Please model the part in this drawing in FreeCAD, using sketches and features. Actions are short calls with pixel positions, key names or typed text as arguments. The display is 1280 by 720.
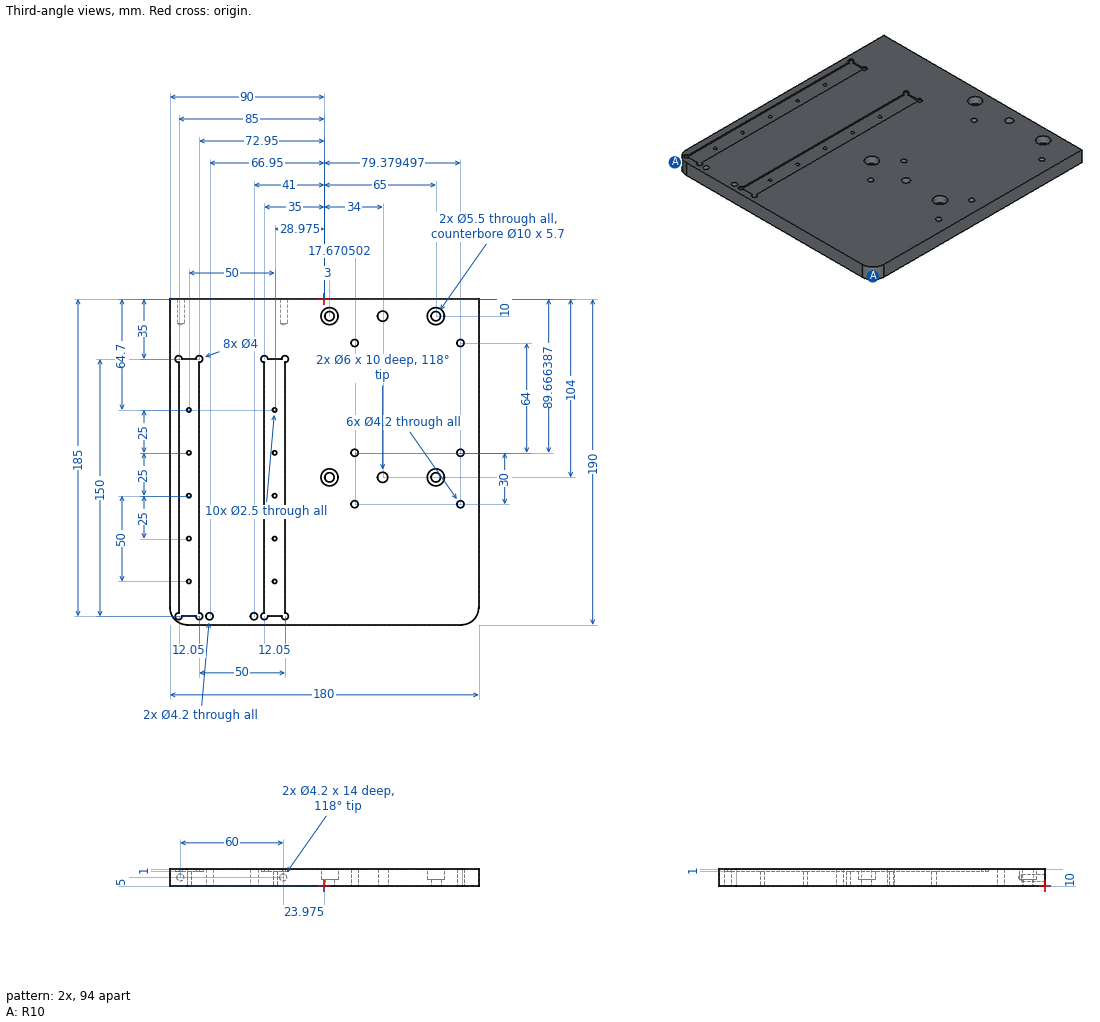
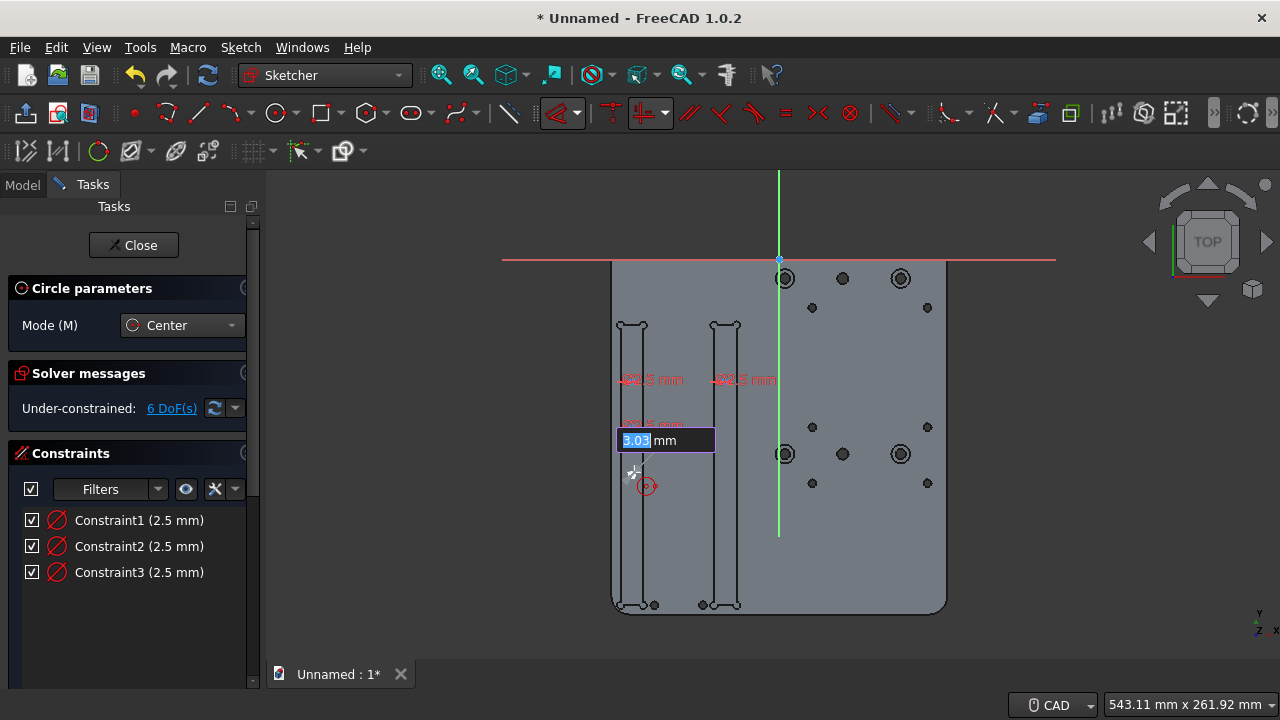
text(2.5)
key(Return)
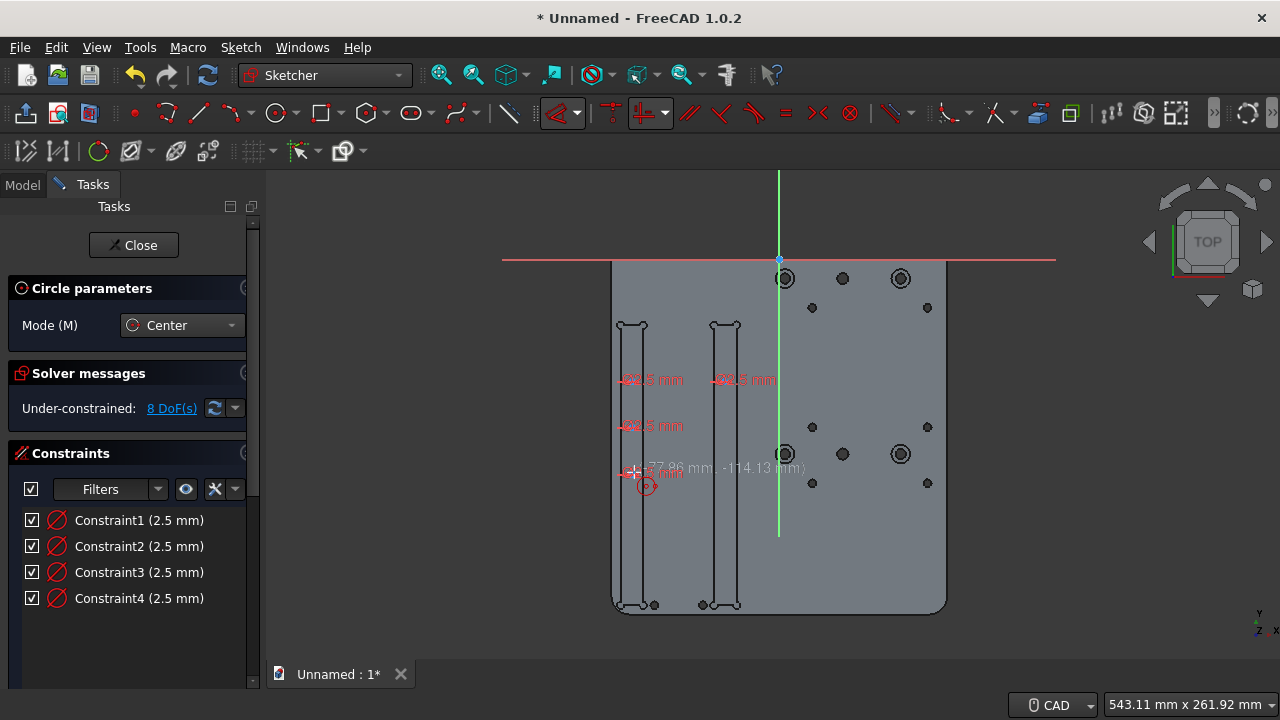
scroll(632, 567, up, 12)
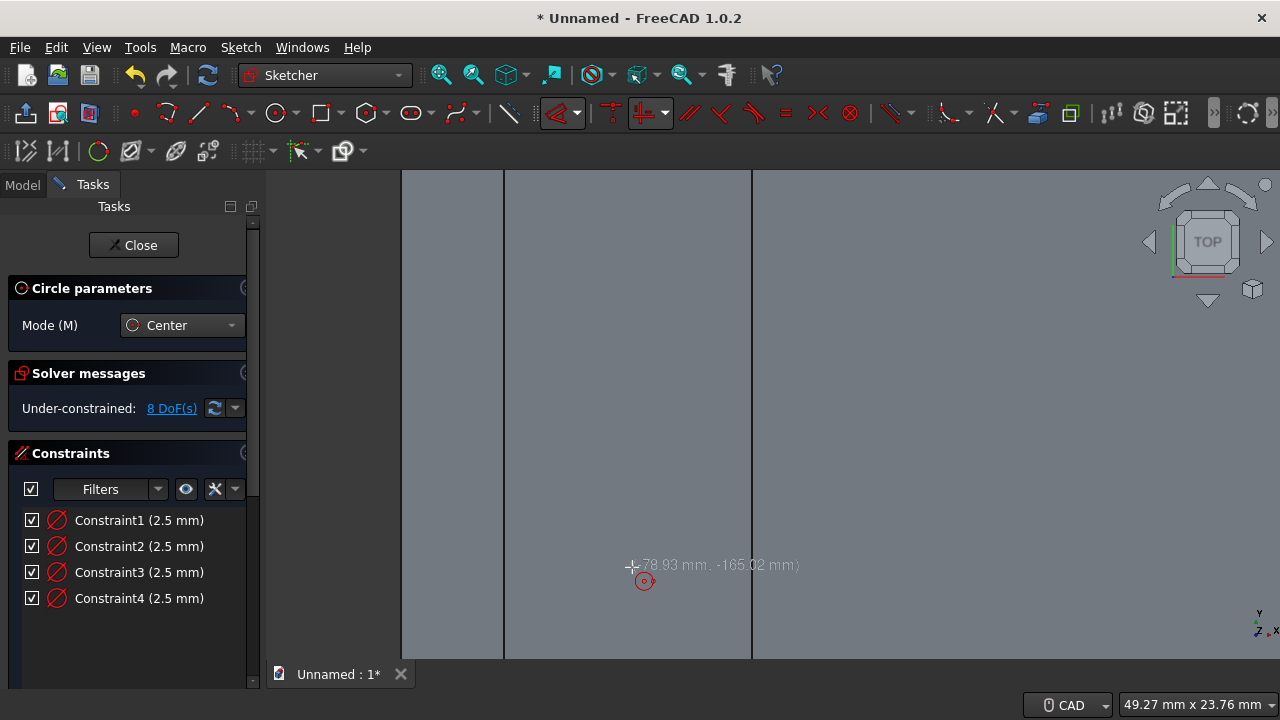
scroll(632, 567, down, 12)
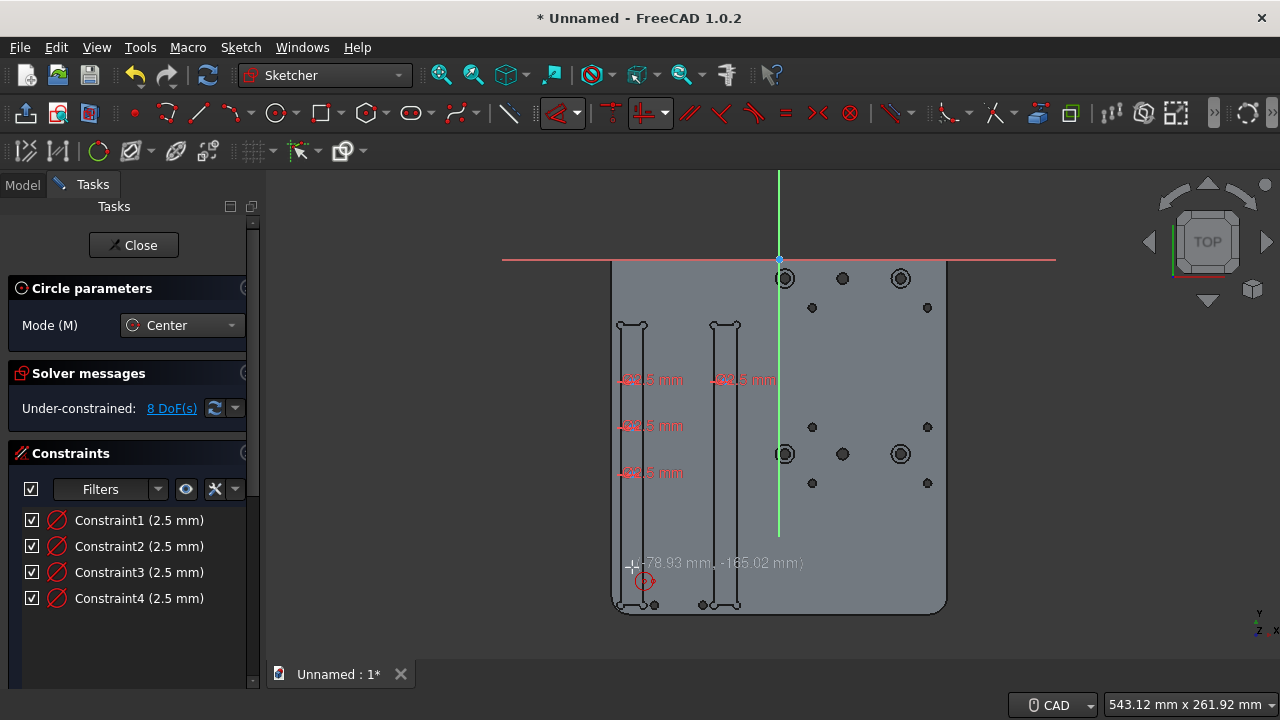
click(632, 567)
move(634, 566)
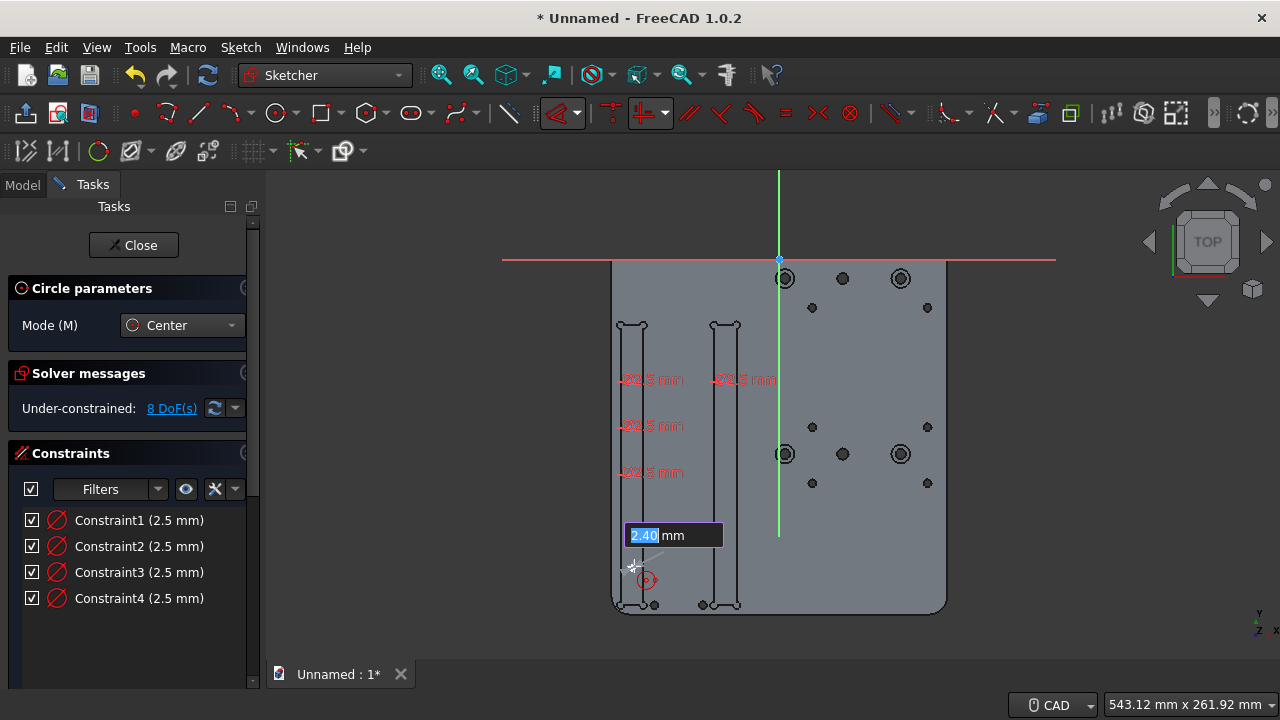
text(2.5)
key(Return)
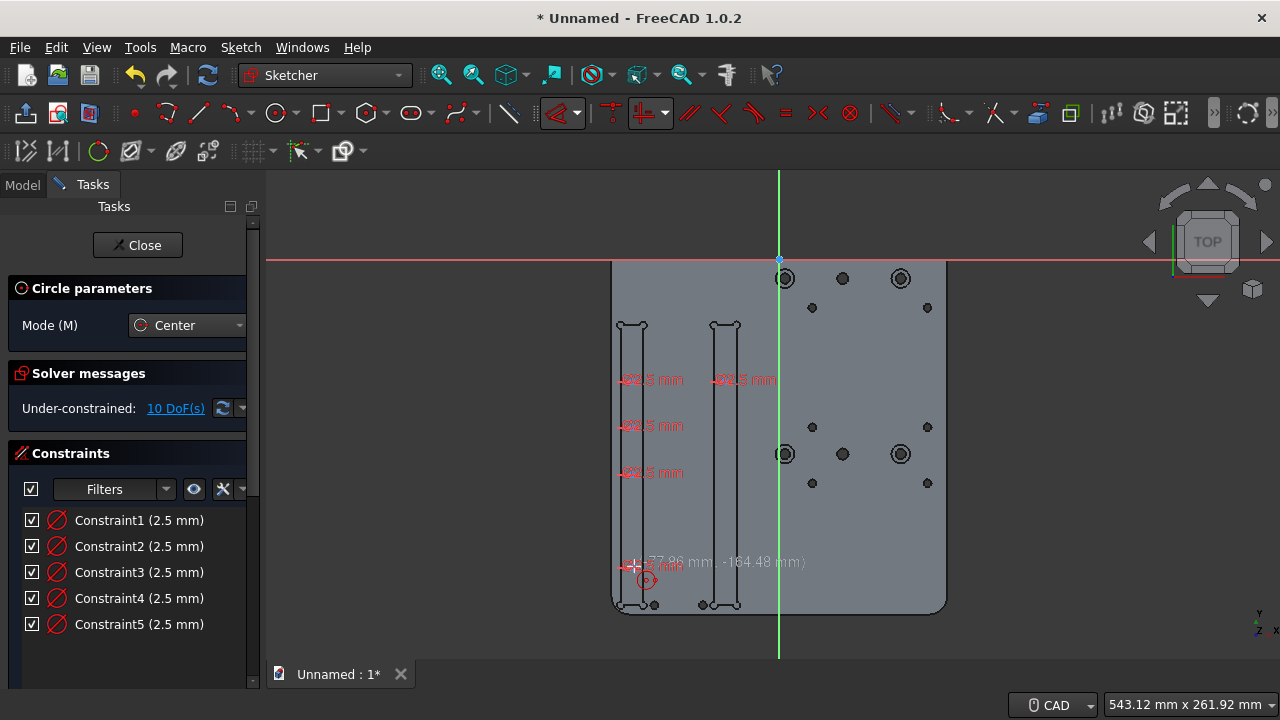
scroll(632, 521, up, 12)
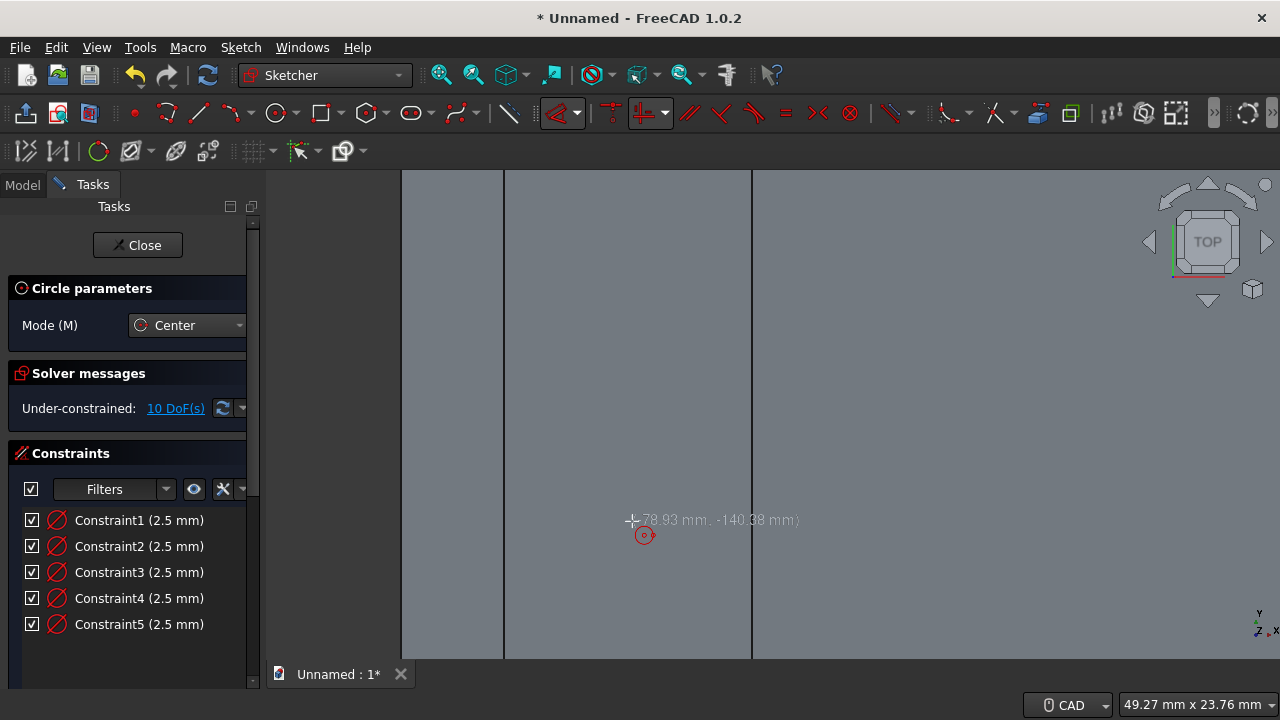
scroll(632, 521, down, 12)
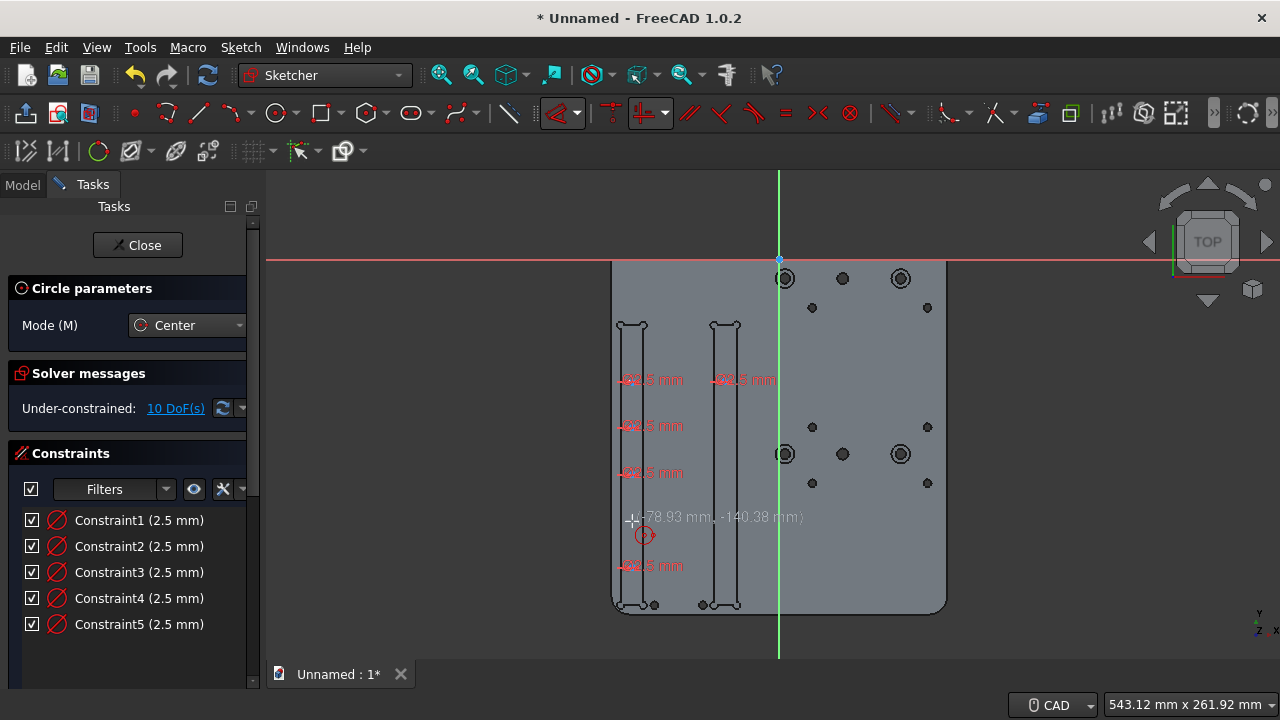
click(632, 521)
move(634, 519)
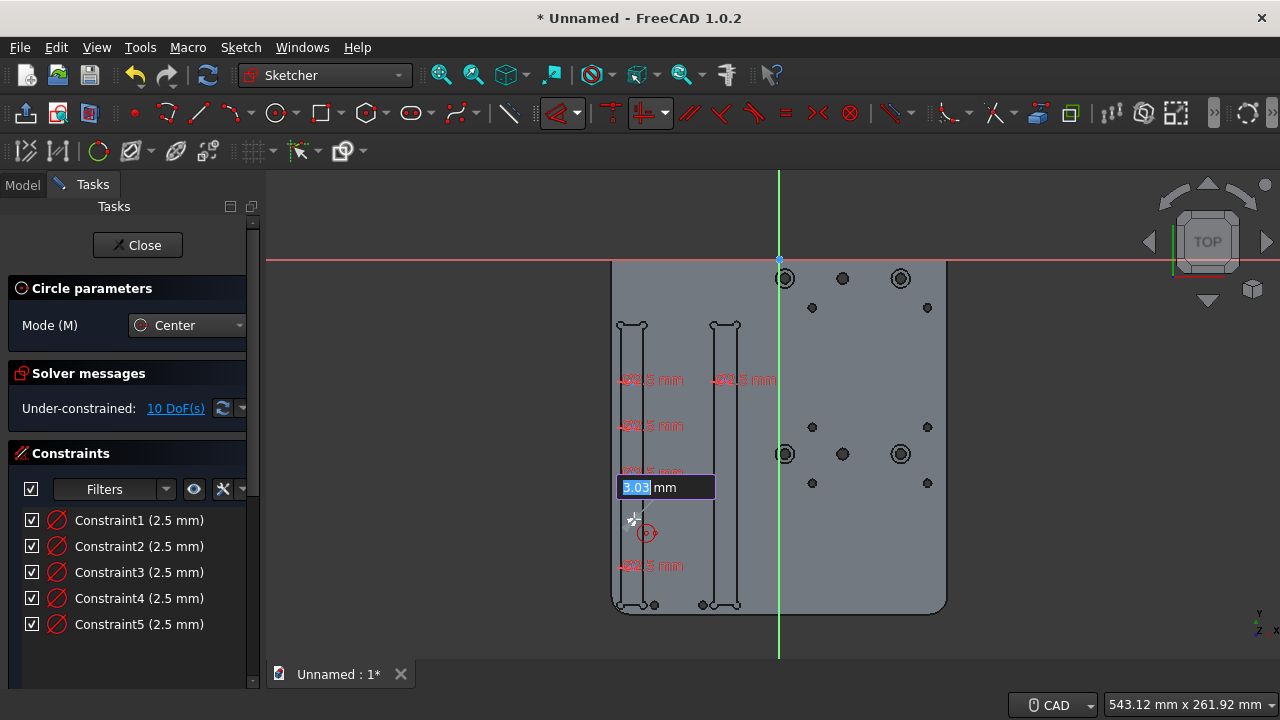
text(2.5)
key(Return)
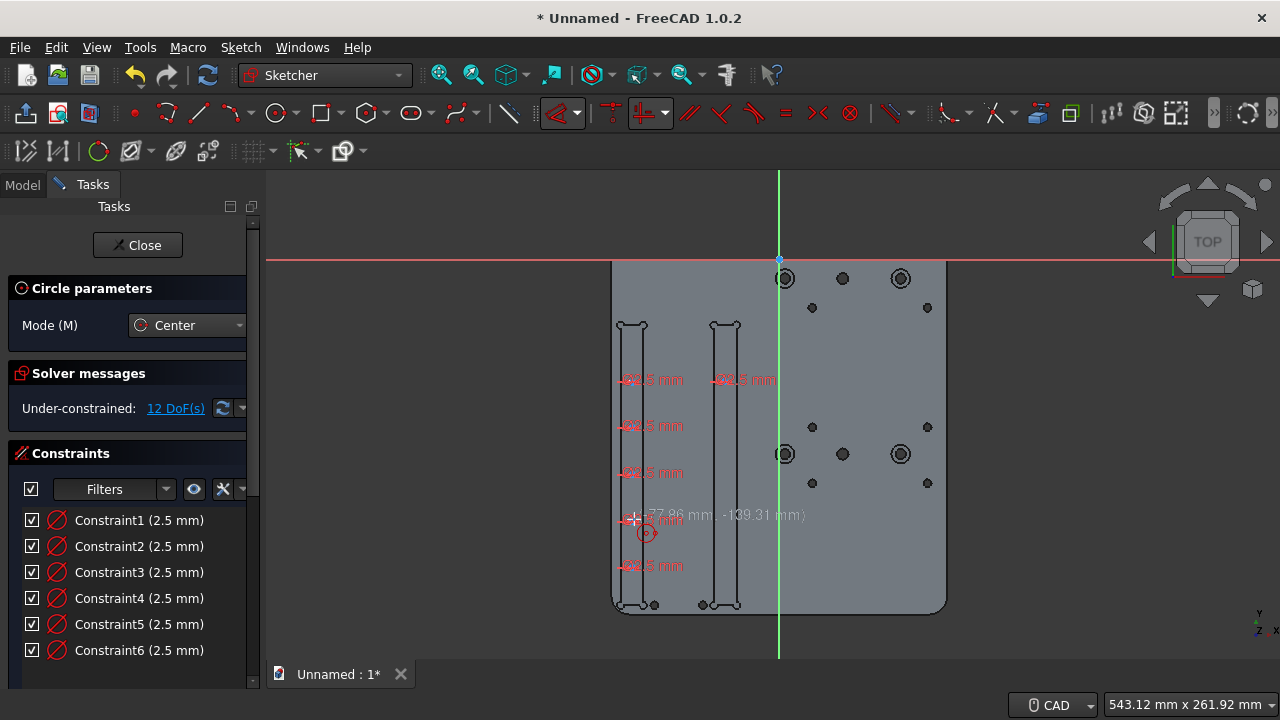
scroll(725, 567, up, 12)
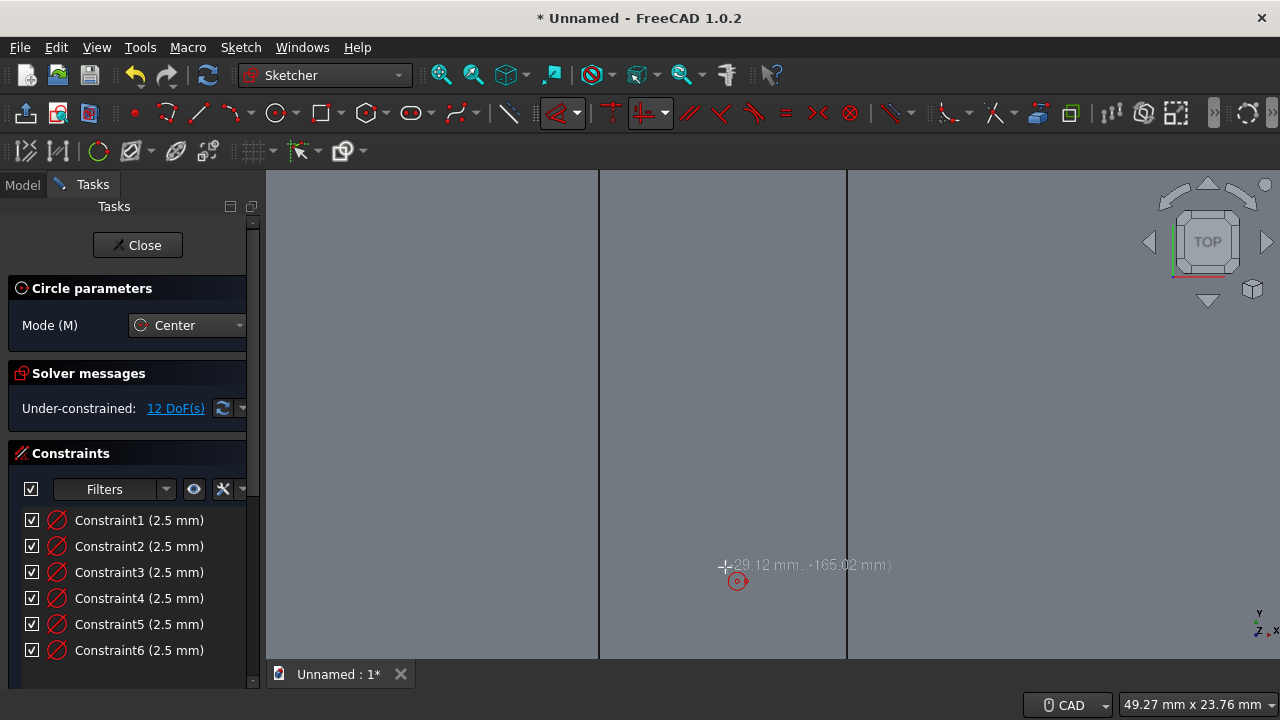
scroll(725, 567, down, 12)